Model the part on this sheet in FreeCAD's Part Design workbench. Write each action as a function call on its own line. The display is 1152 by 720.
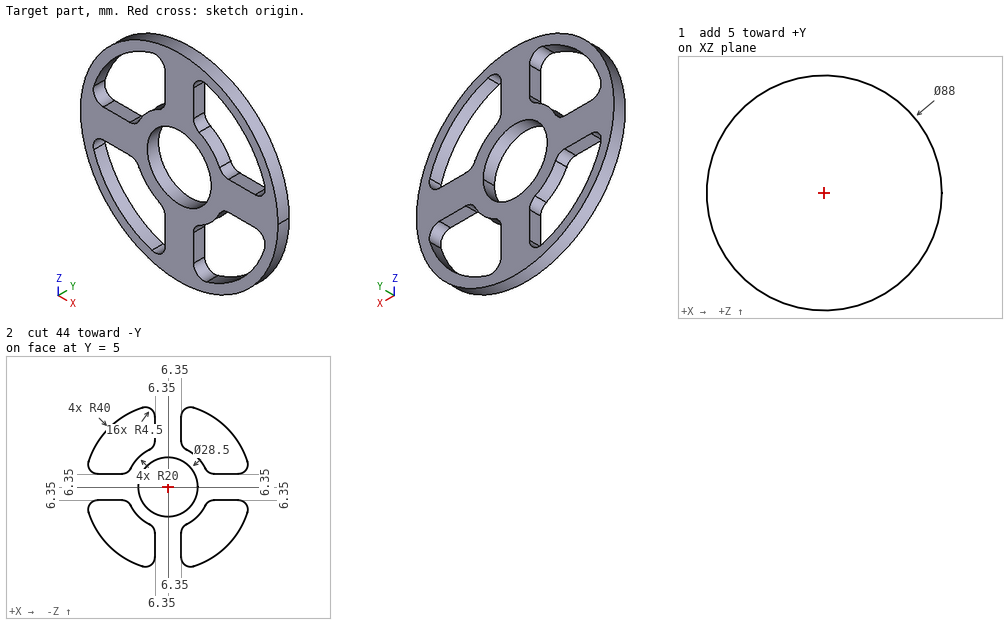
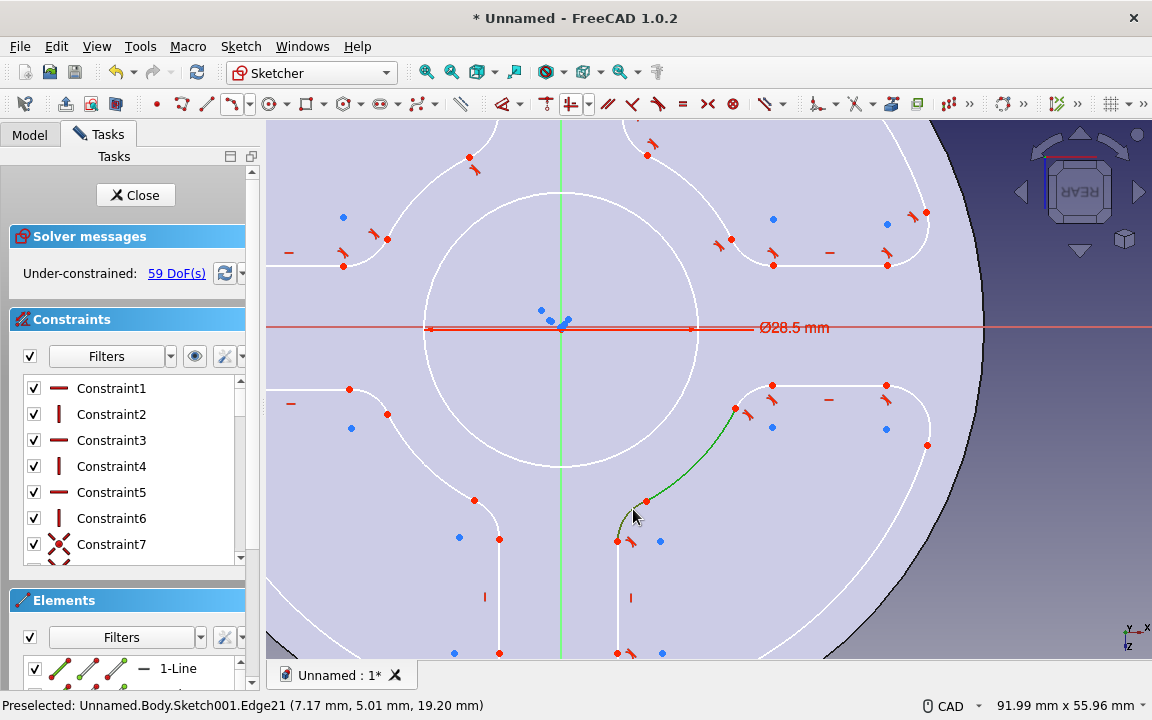
key(t)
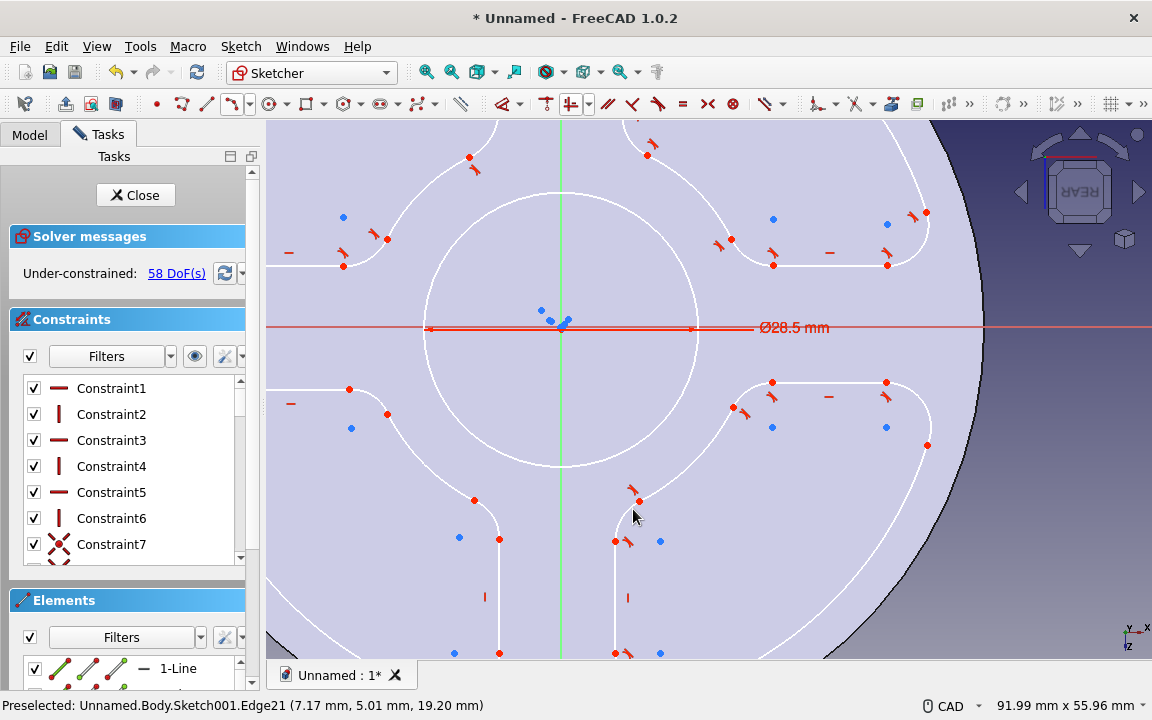
scroll(706, 440, down, 4)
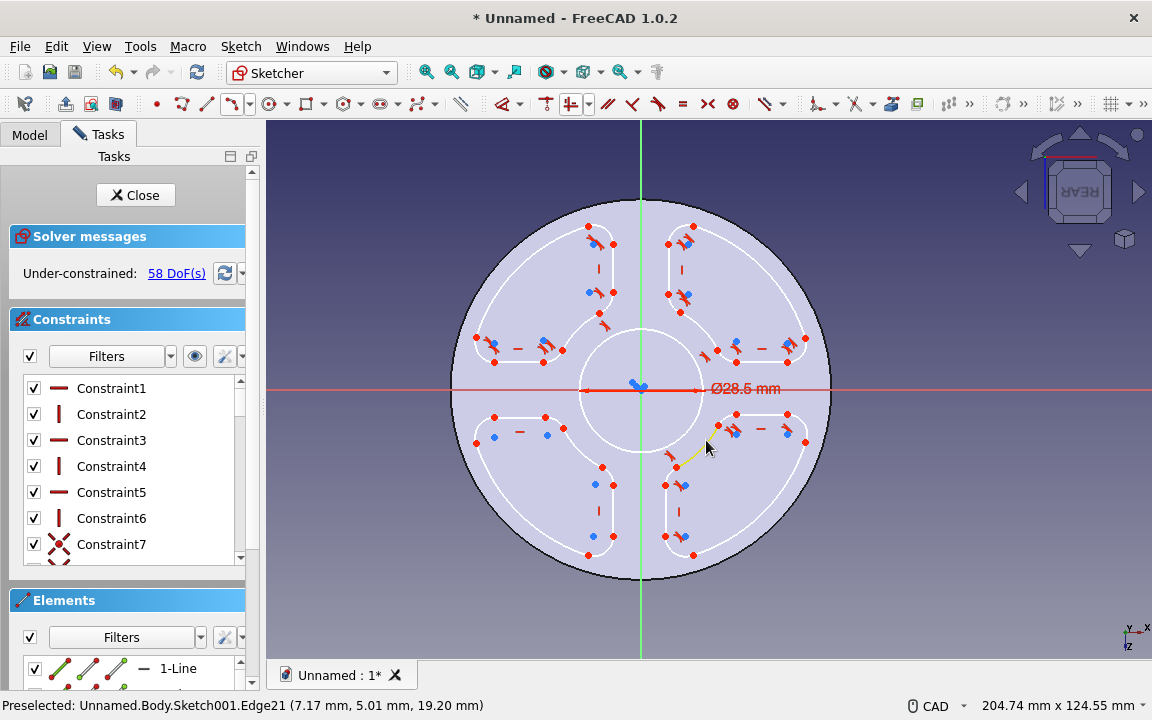
click(669, 548)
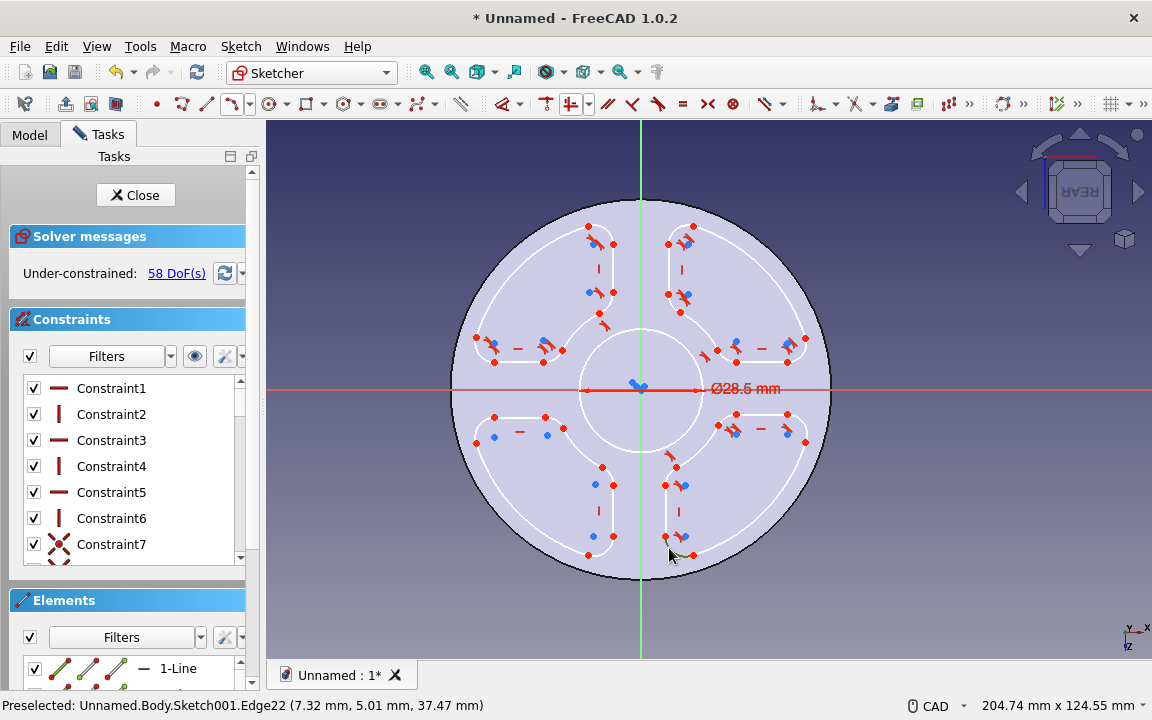
click(738, 534)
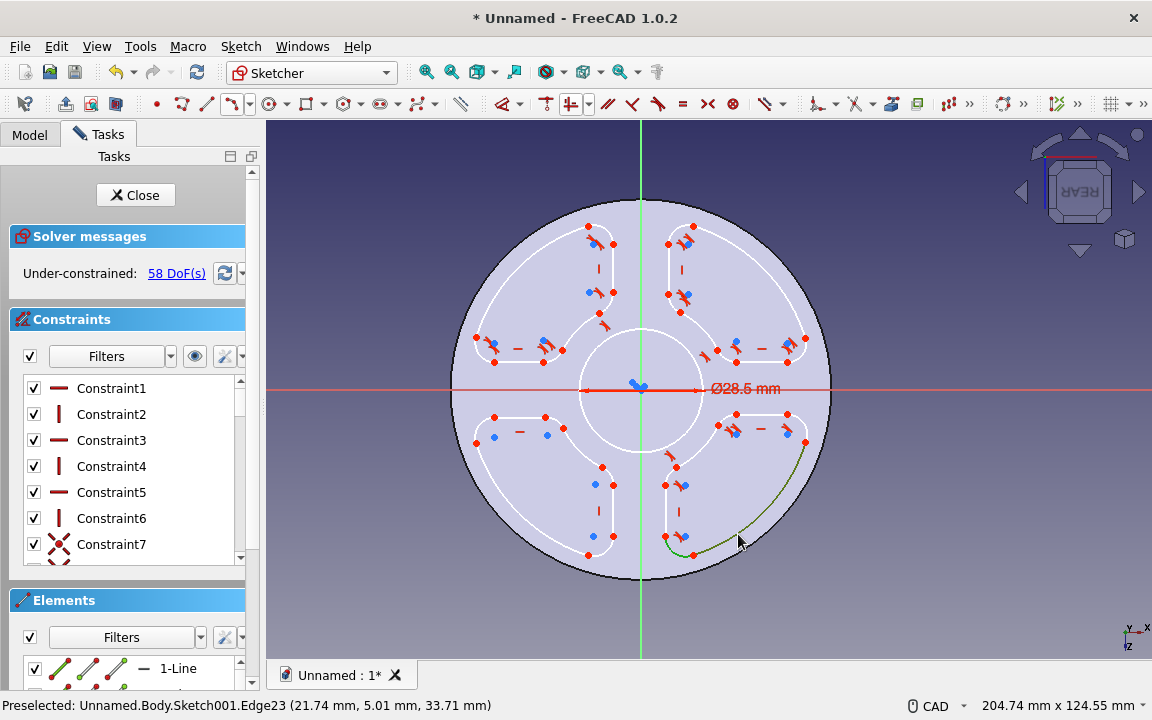
key(t)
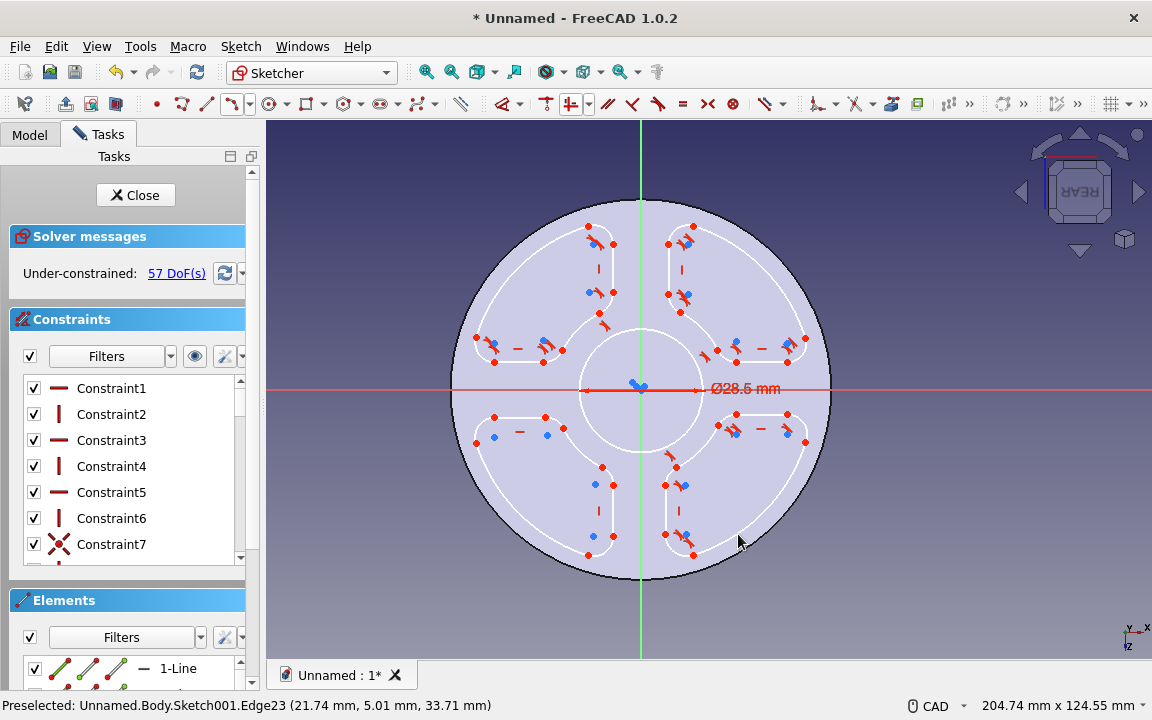
click(738, 534)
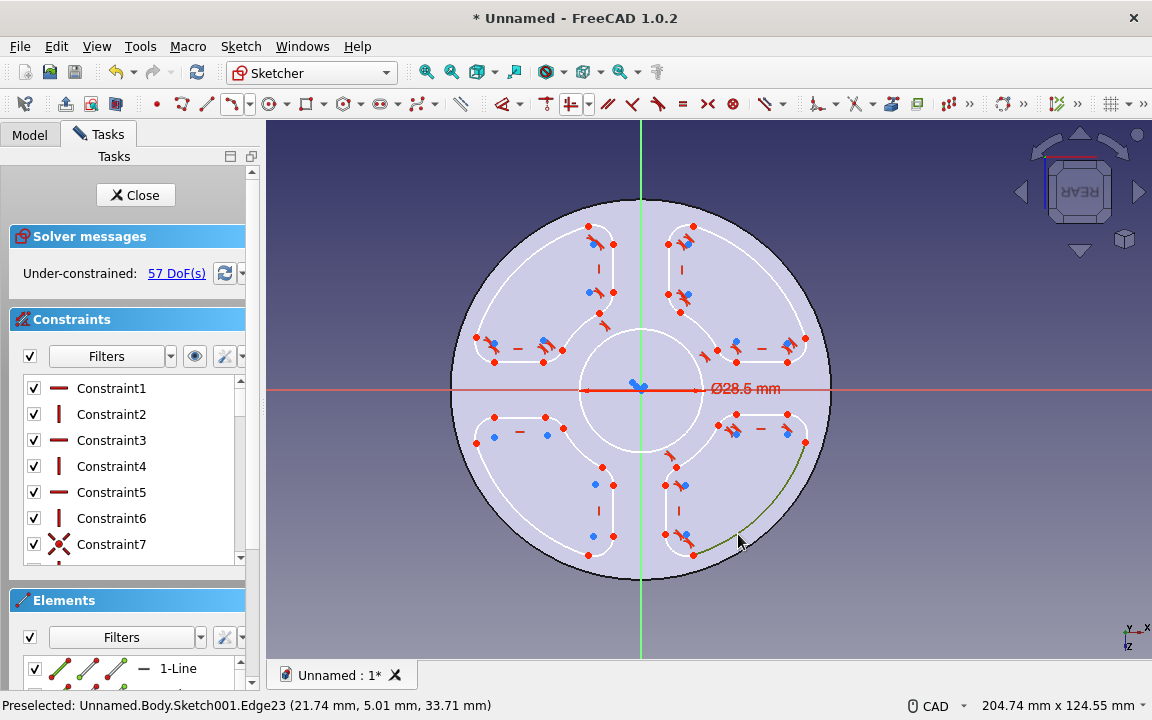
click(807, 431)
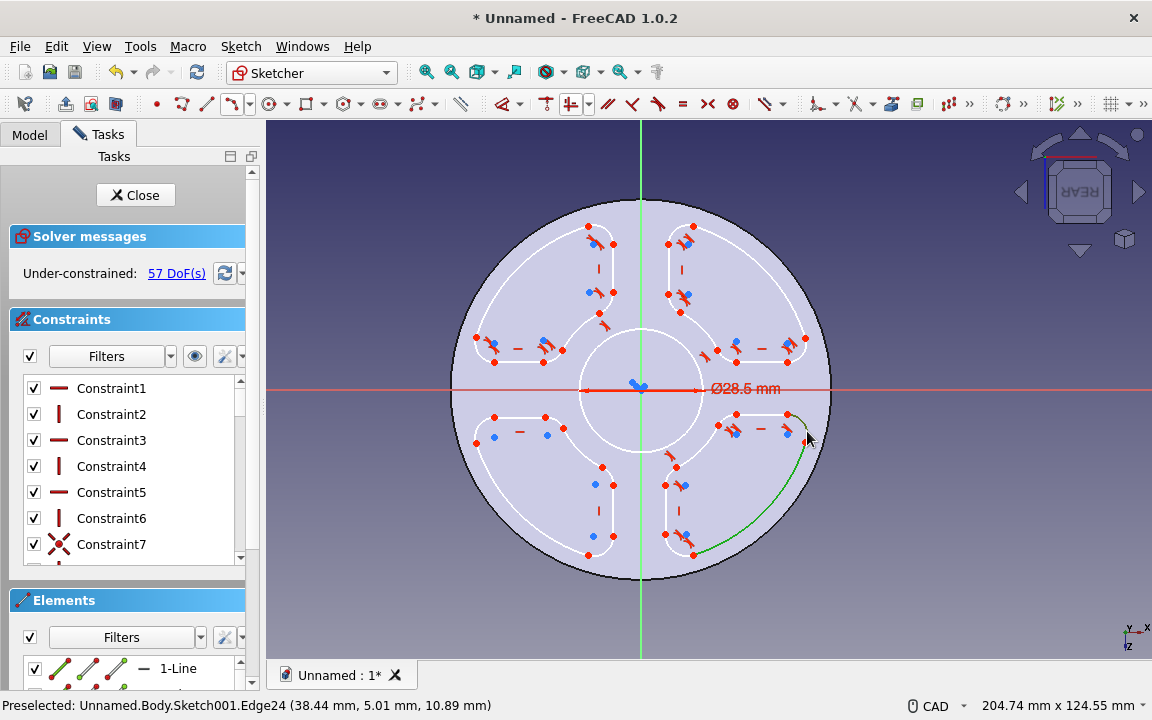
key(t)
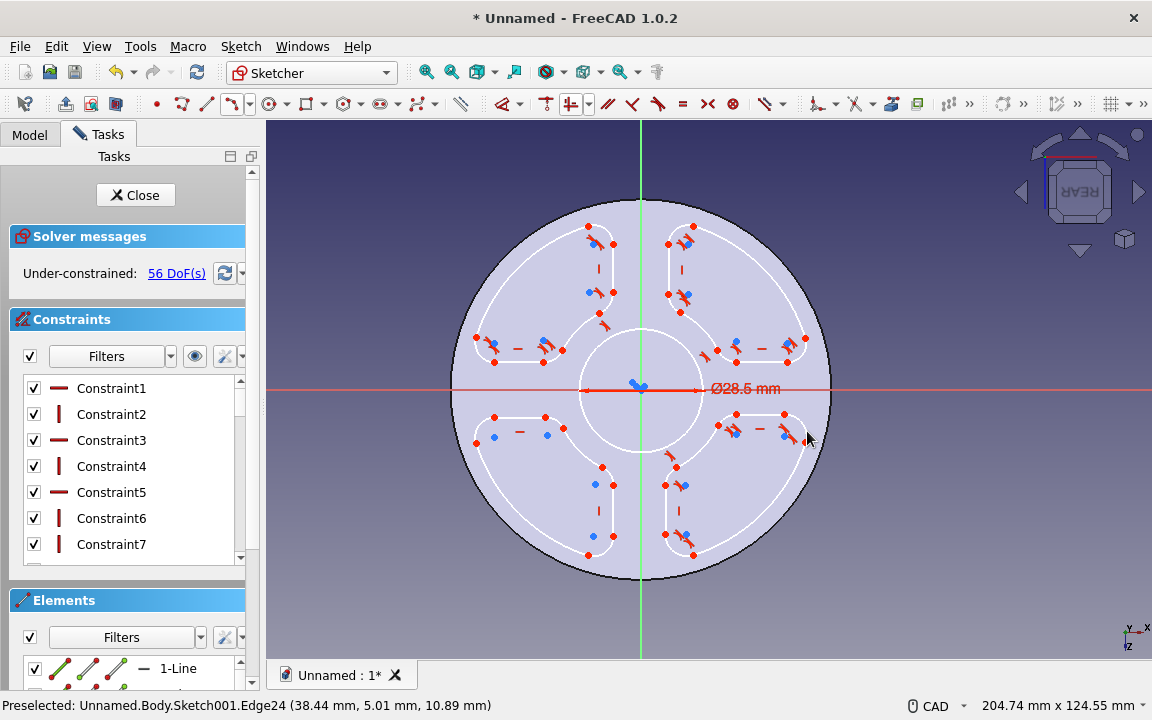
click(613, 521)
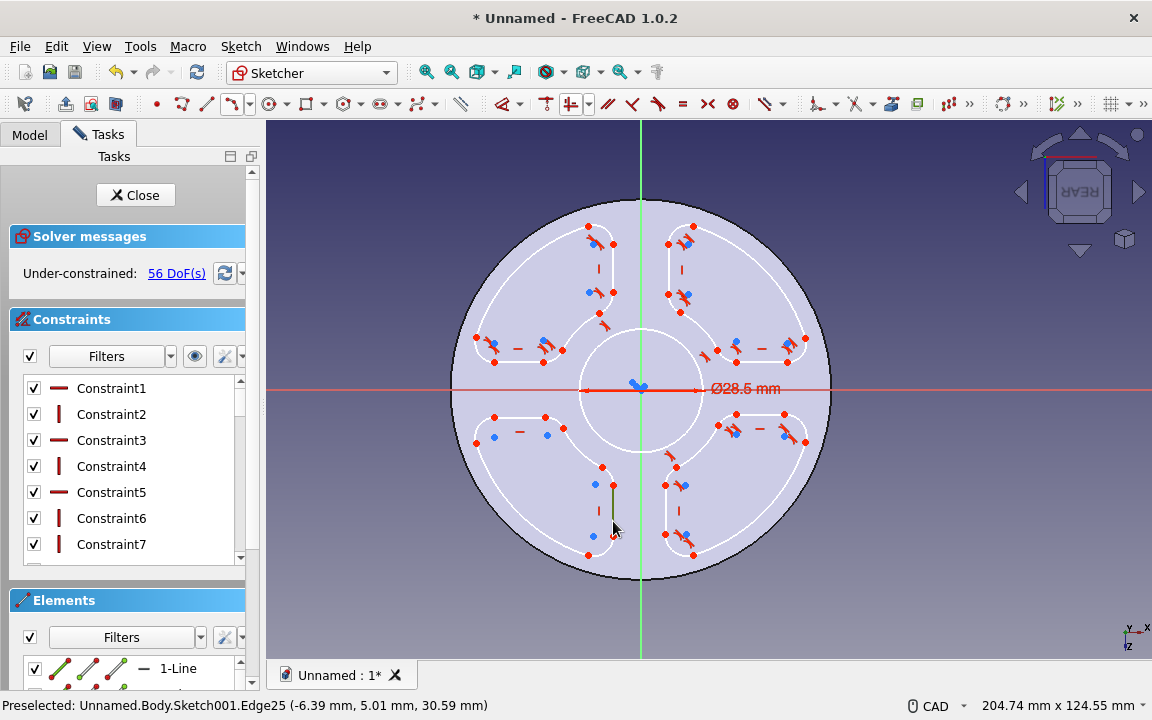
scroll(611, 475, up, 2)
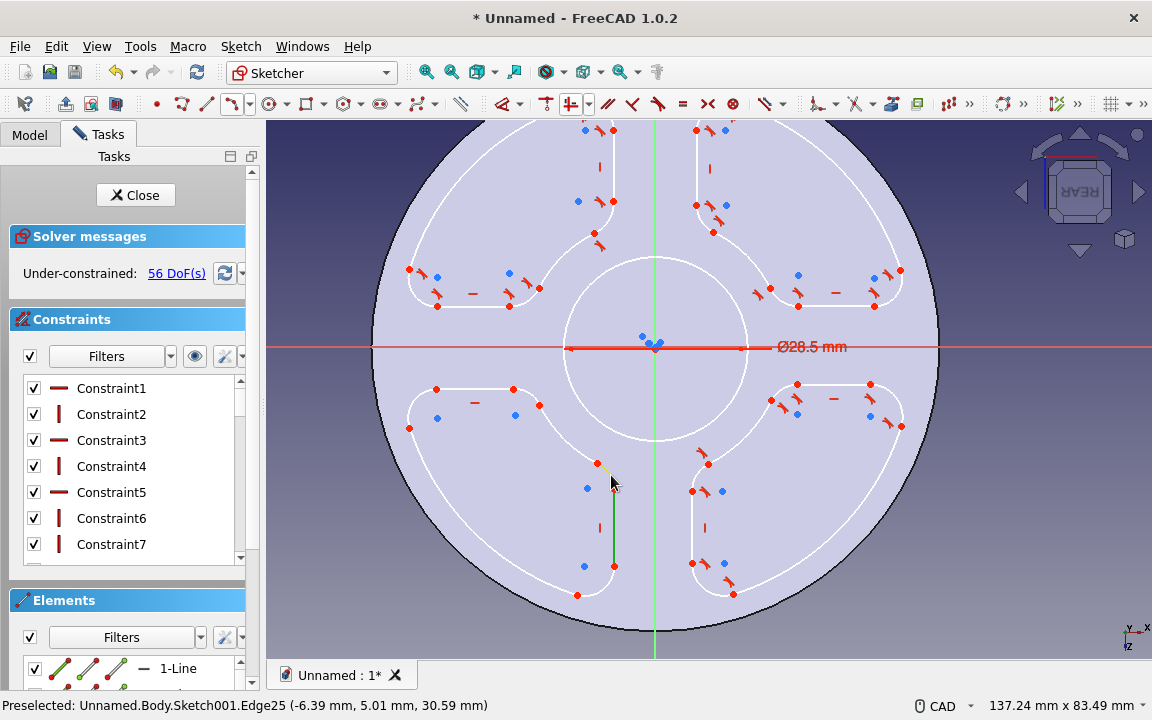
click(610, 474)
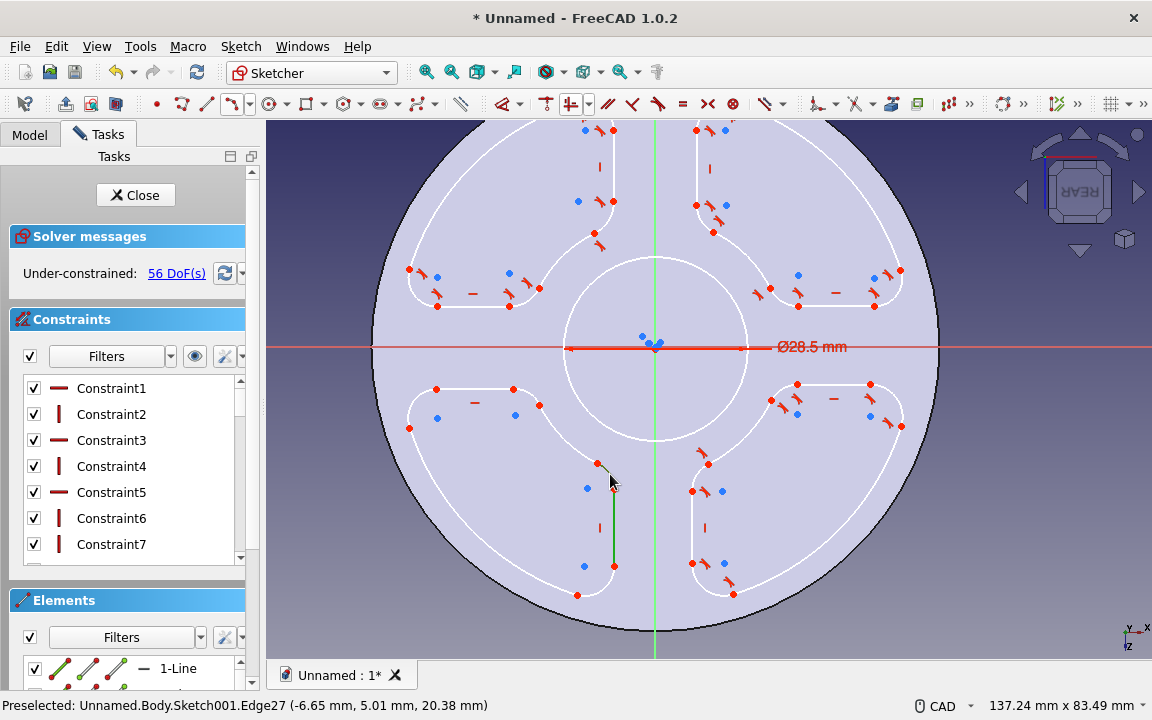
key(t)